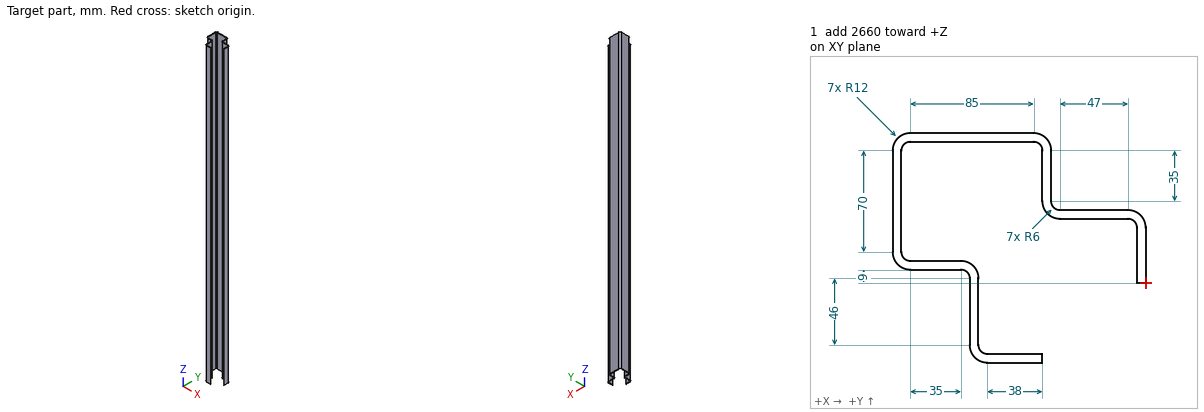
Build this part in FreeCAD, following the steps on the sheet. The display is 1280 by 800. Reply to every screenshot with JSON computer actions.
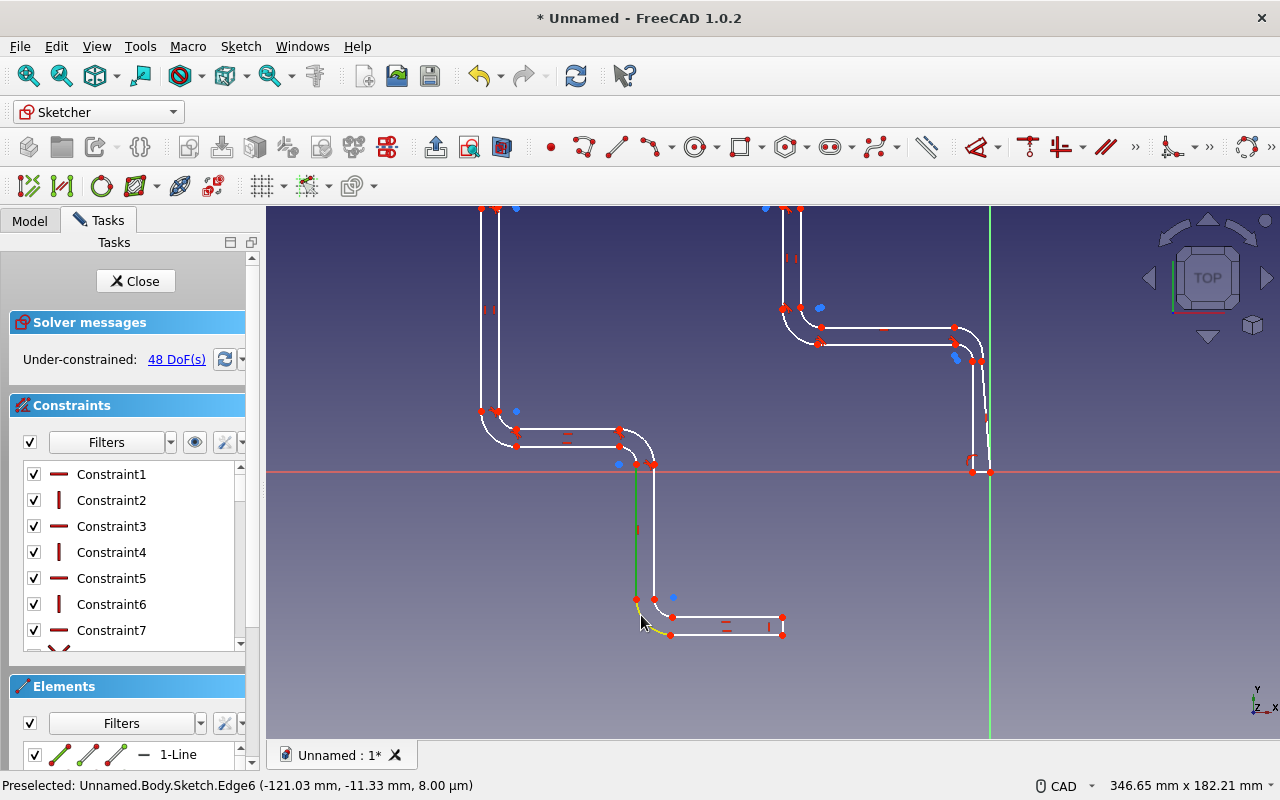
{"action": "left_click", "coordinate": [641, 615]}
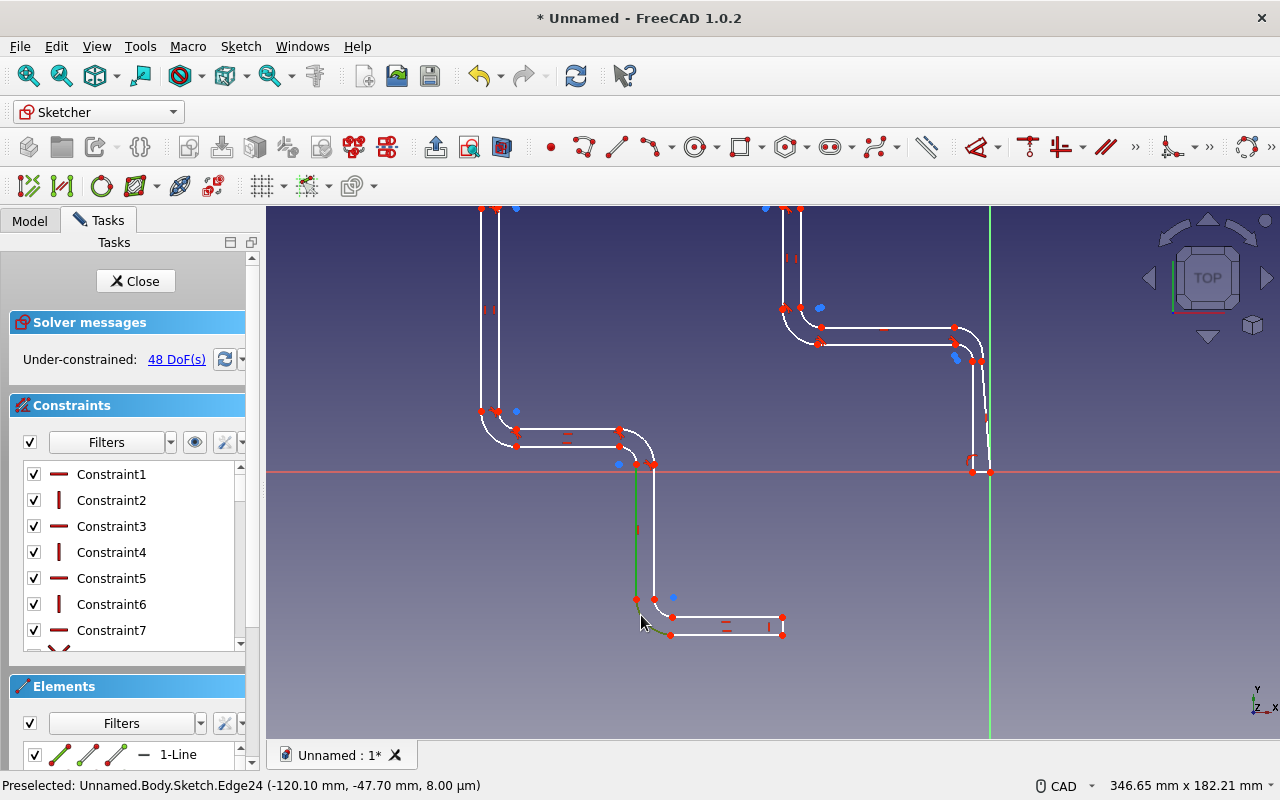
{"action": "key", "text": "t"}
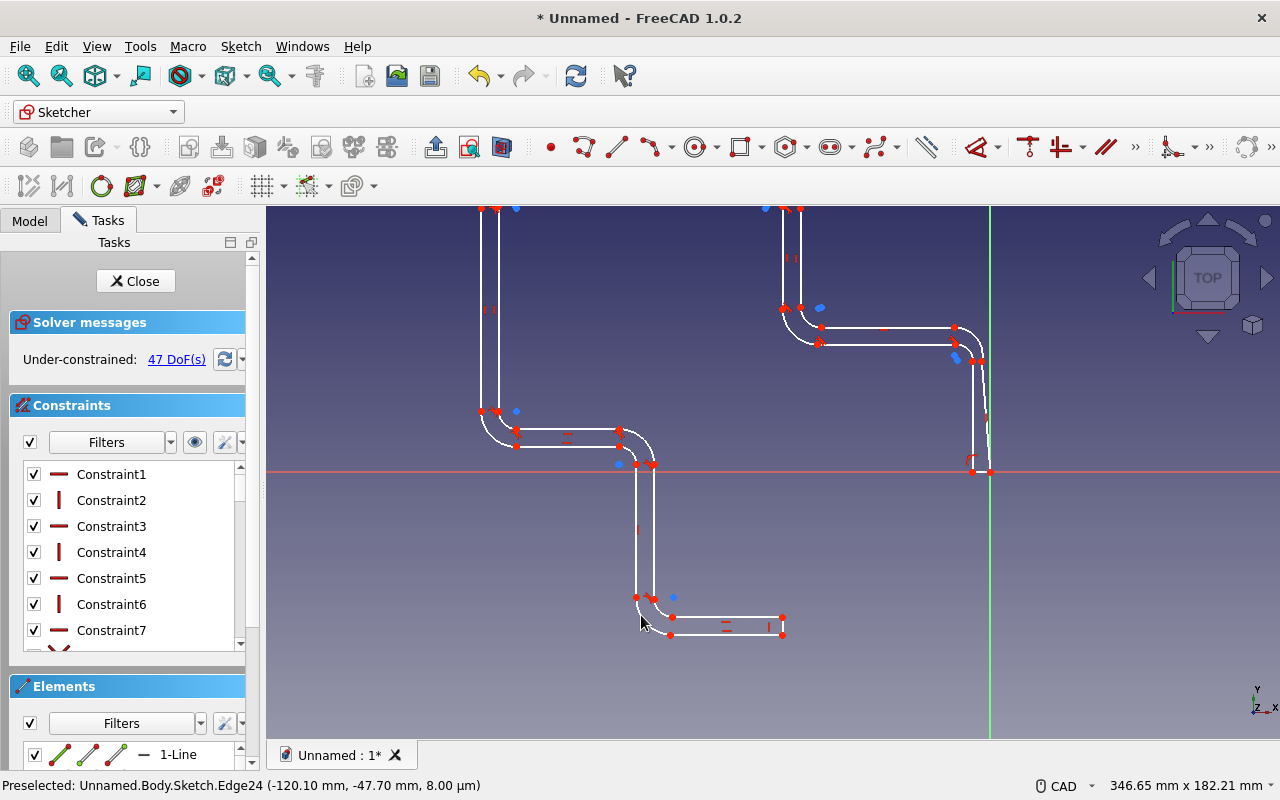
{"action": "left_click", "coordinate": [705, 635]}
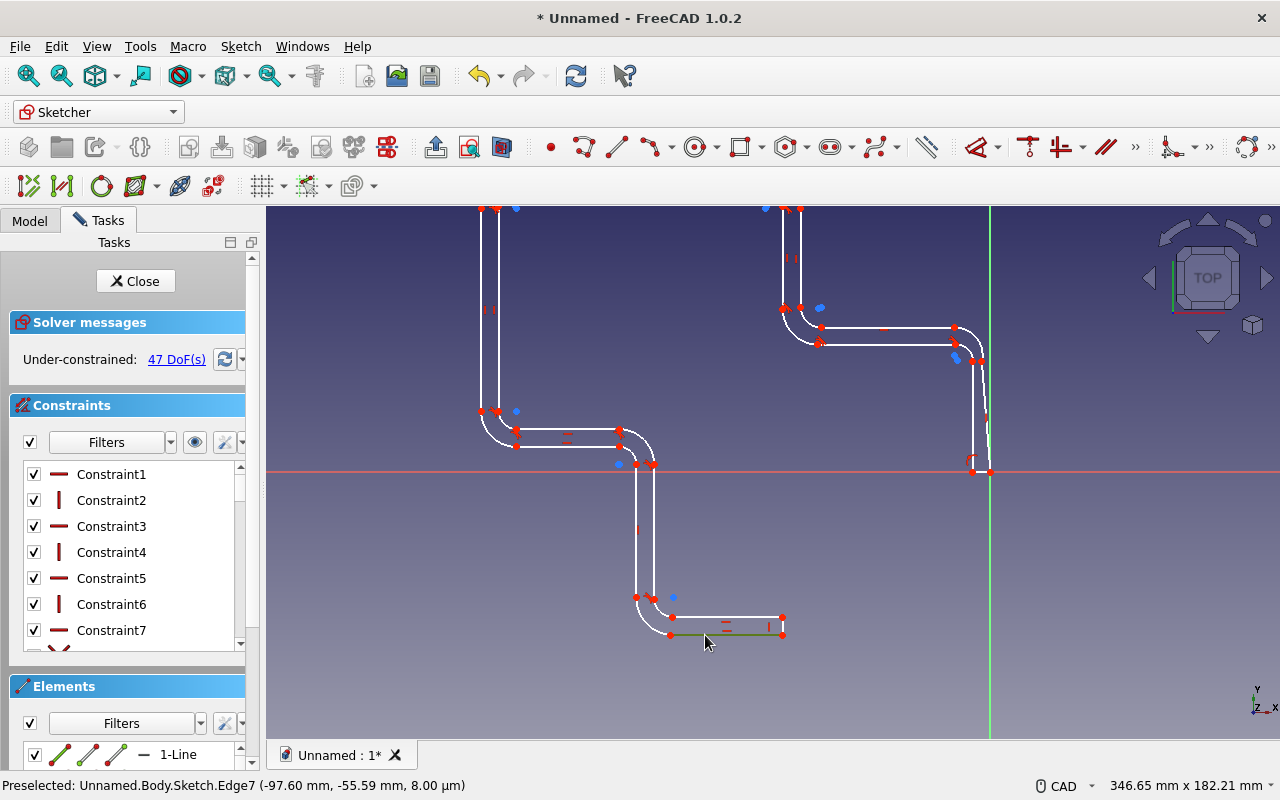
{"action": "left_click", "coordinate": [640, 614]}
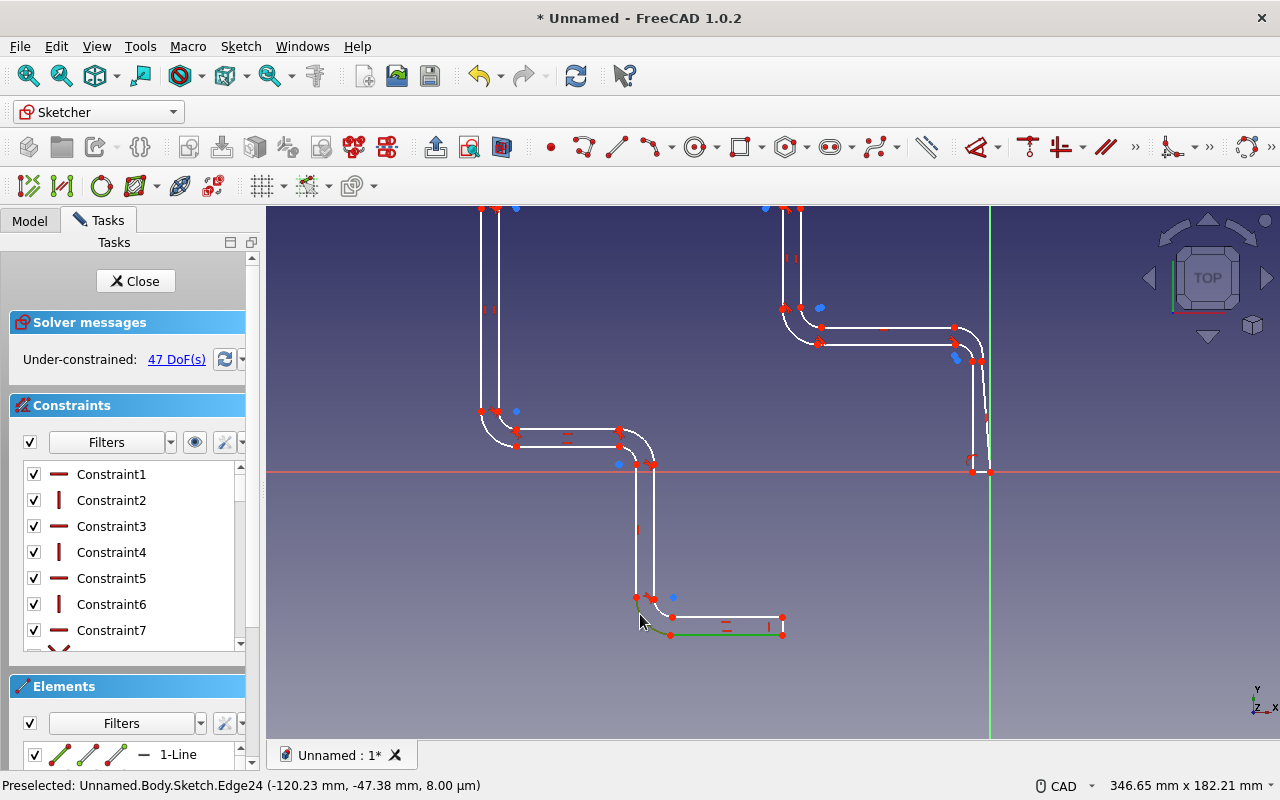
{"action": "key", "text": "t"}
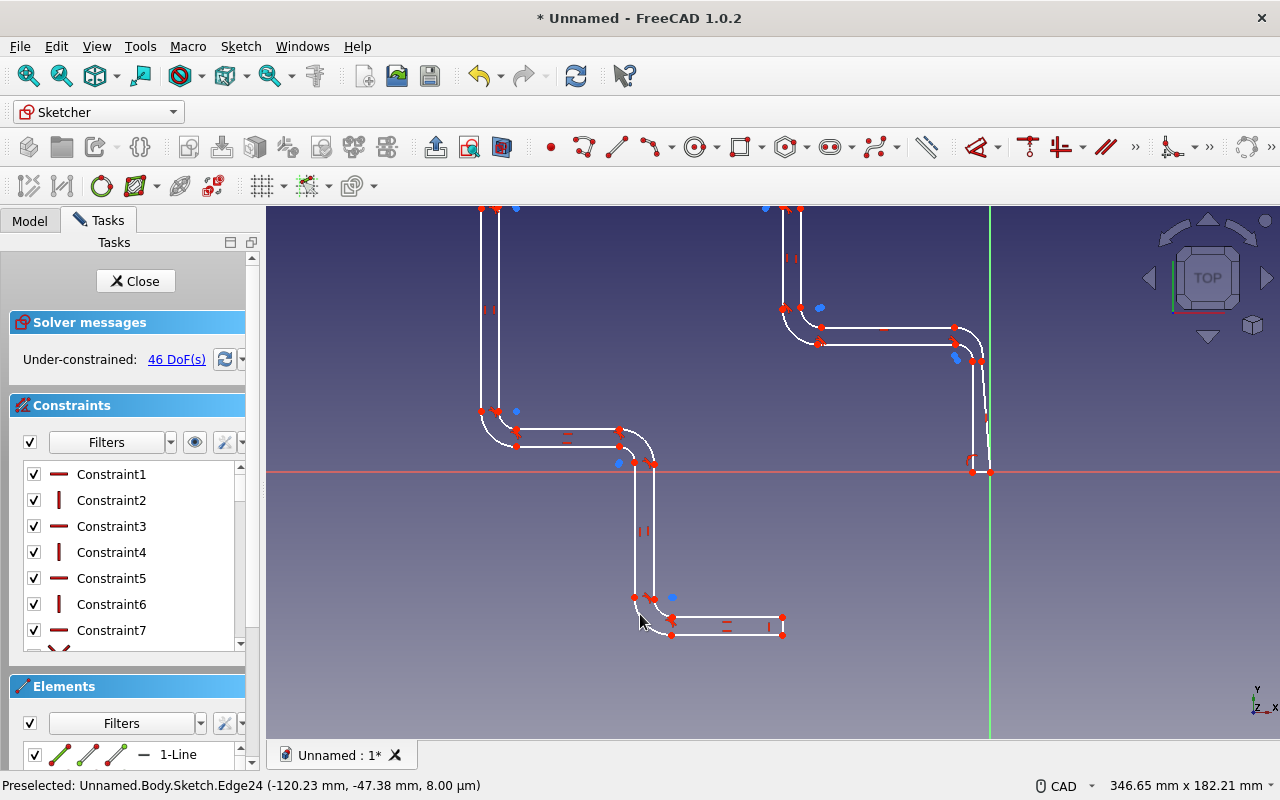
{"action": "left_click", "coordinate": [750, 617]}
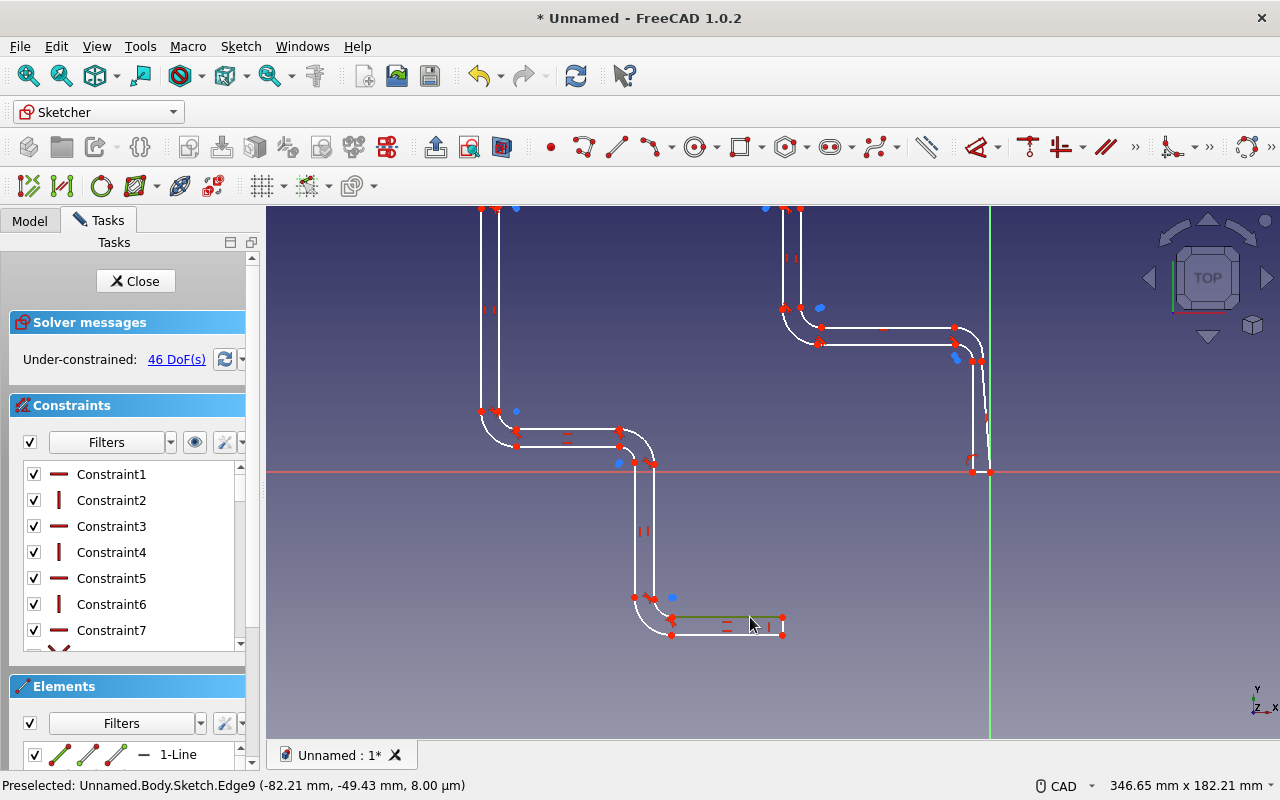
{"action": "left_click", "coordinate": [660, 611]}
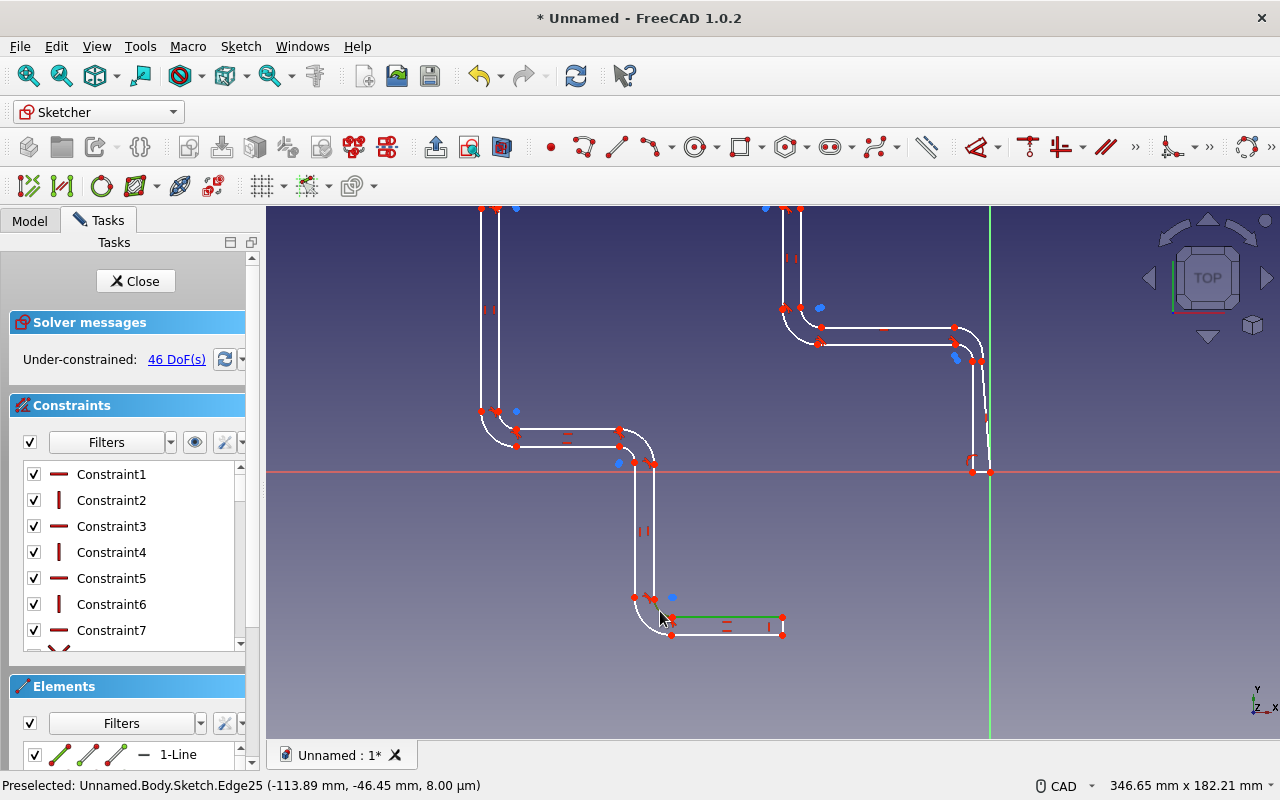
{"action": "key", "text": "t"}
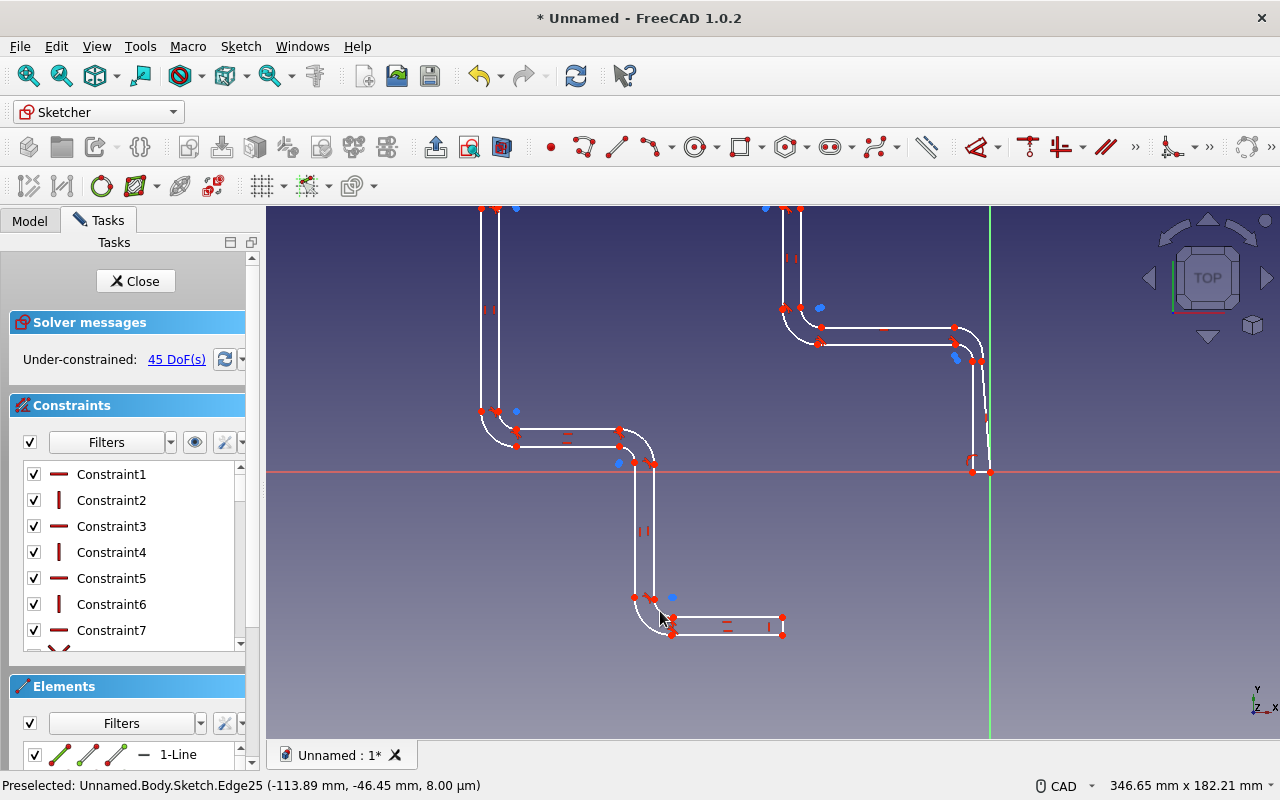
{"action": "left_click", "coordinate": [654, 559]}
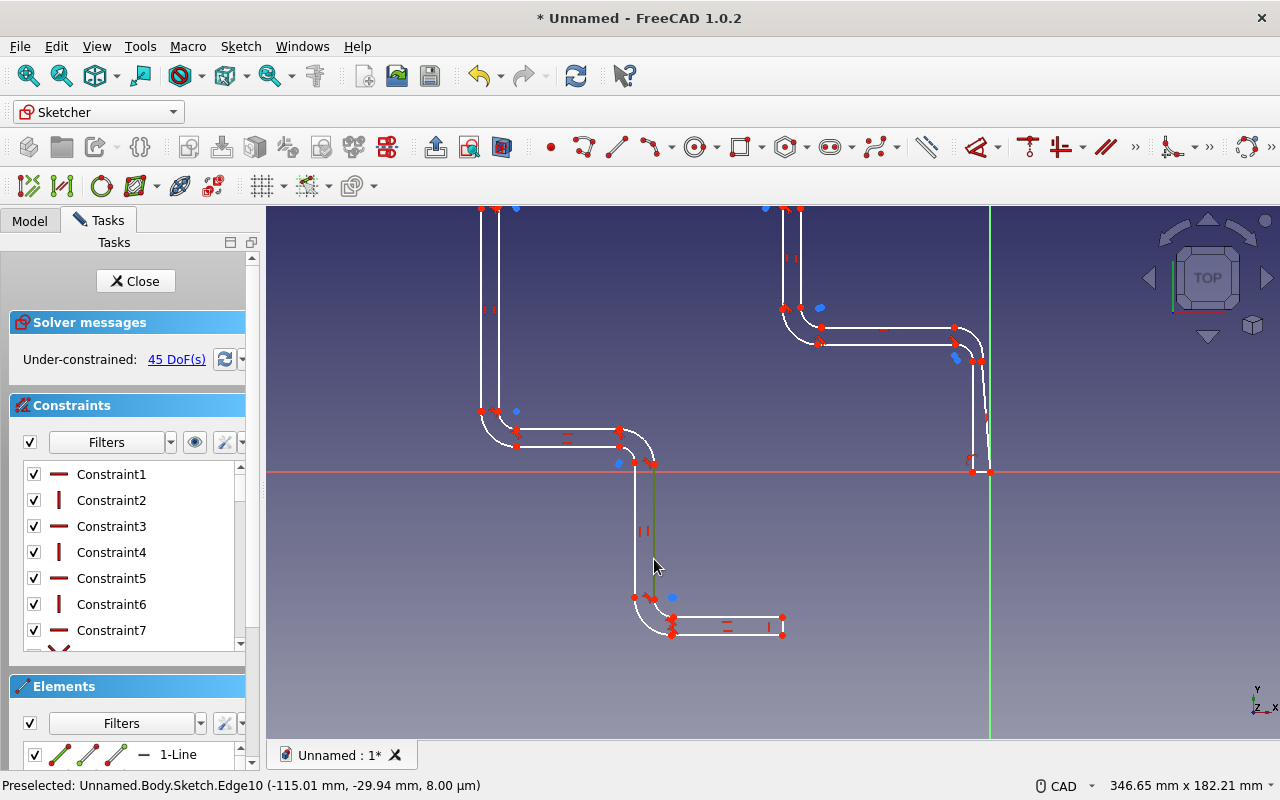
{"action": "left_click", "coordinate": [660, 612]}